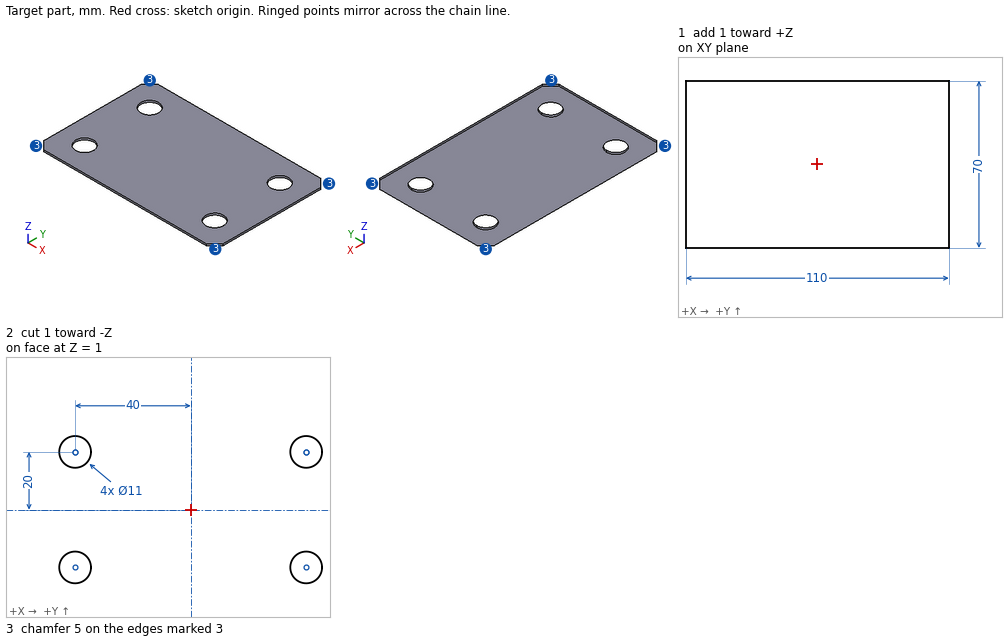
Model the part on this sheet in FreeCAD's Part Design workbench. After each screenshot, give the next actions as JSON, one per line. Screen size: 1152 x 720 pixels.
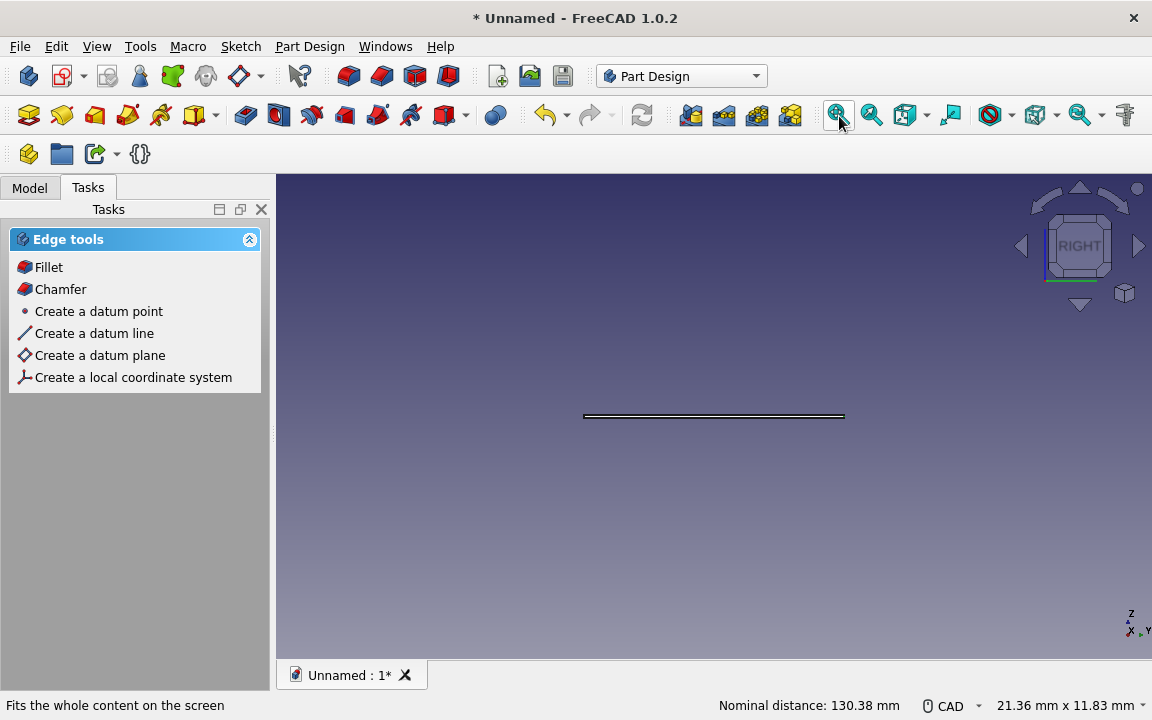
{"action": "key", "text": "5"}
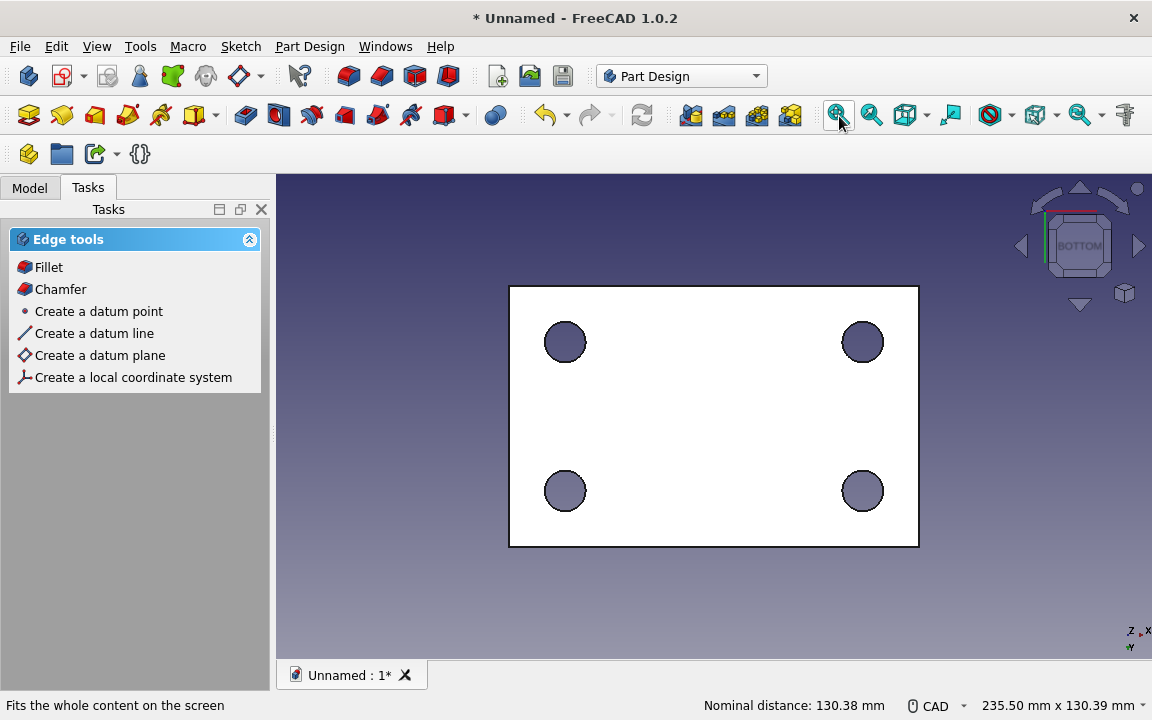
{"action": "scroll", "coordinate": [509, 546], "scroll_direction": "up", "scroll_amount": 12}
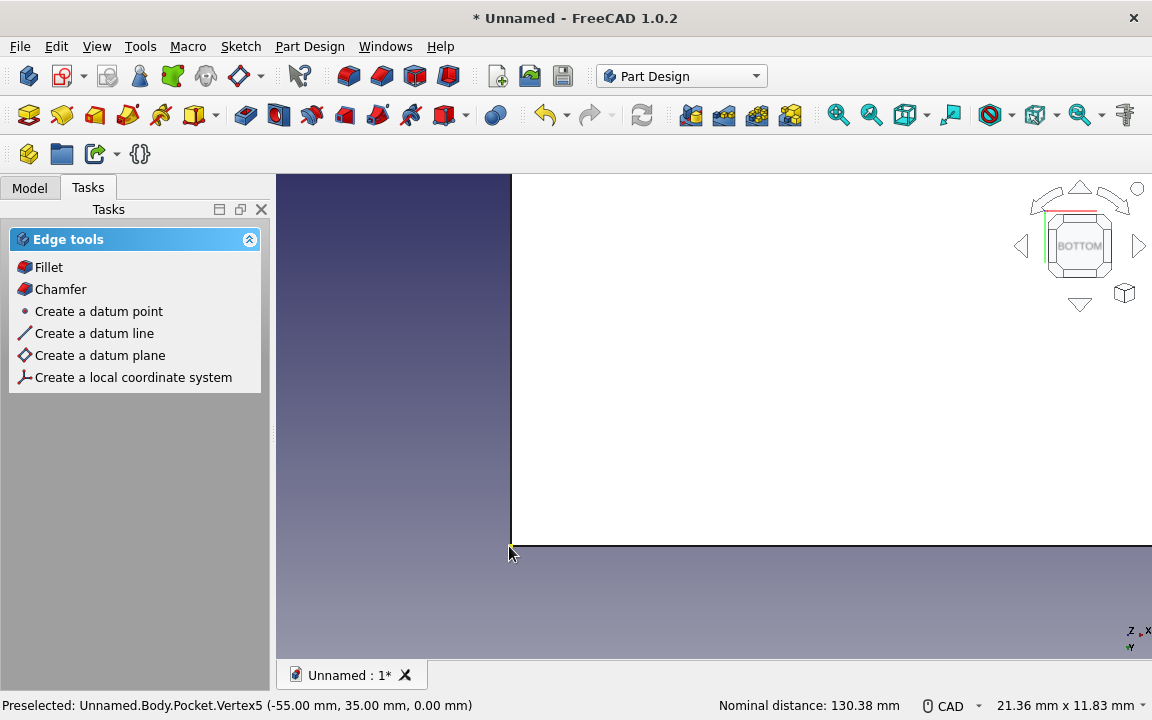
{"action": "left_click", "coordinate": [839, 116]}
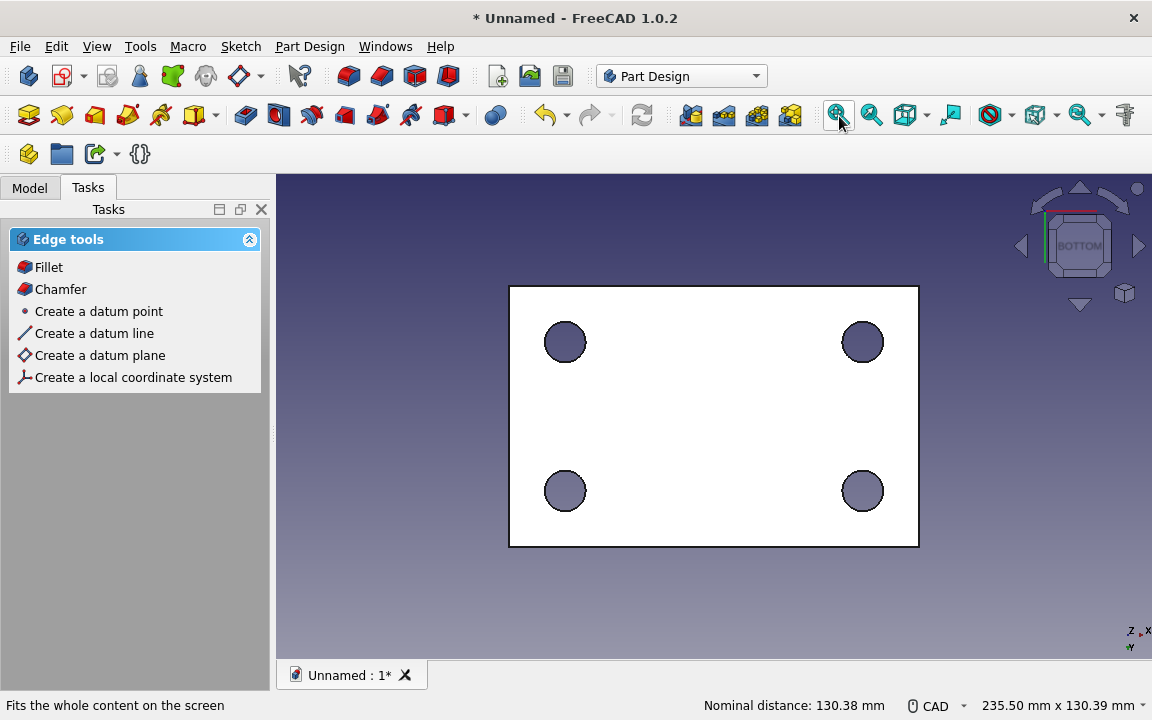
{"action": "key", "text": "4"}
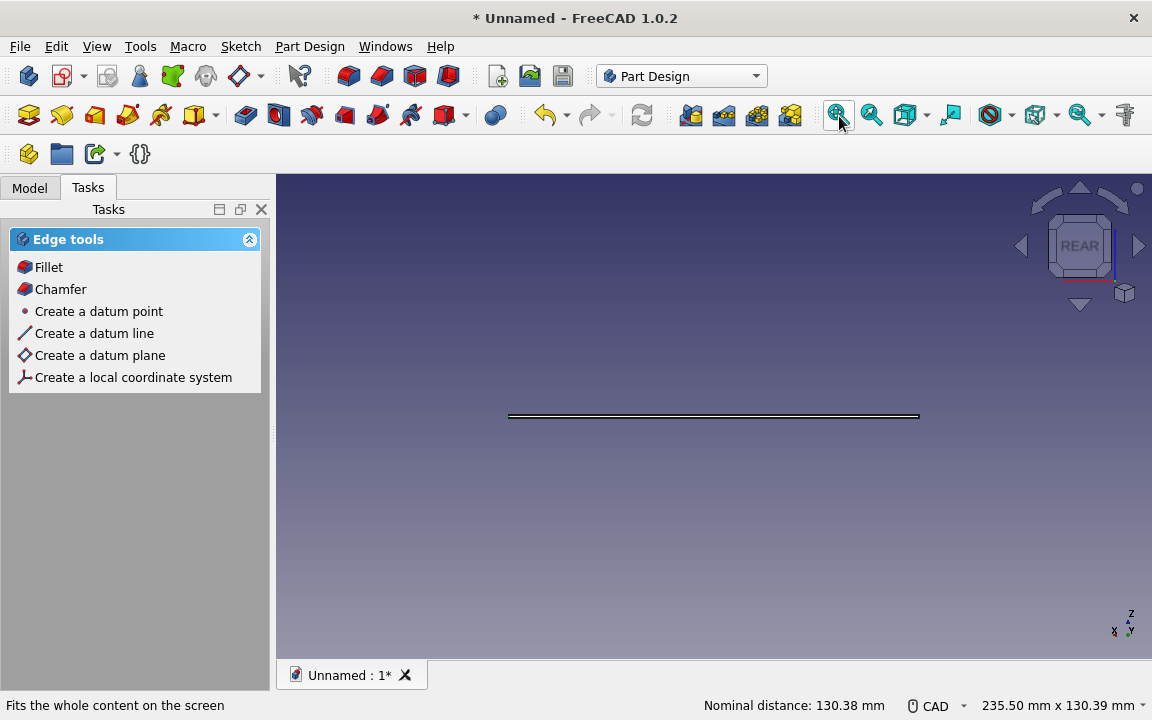
{"action": "scroll", "coordinate": [919, 415], "scroll_direction": "up", "scroll_amount": 12}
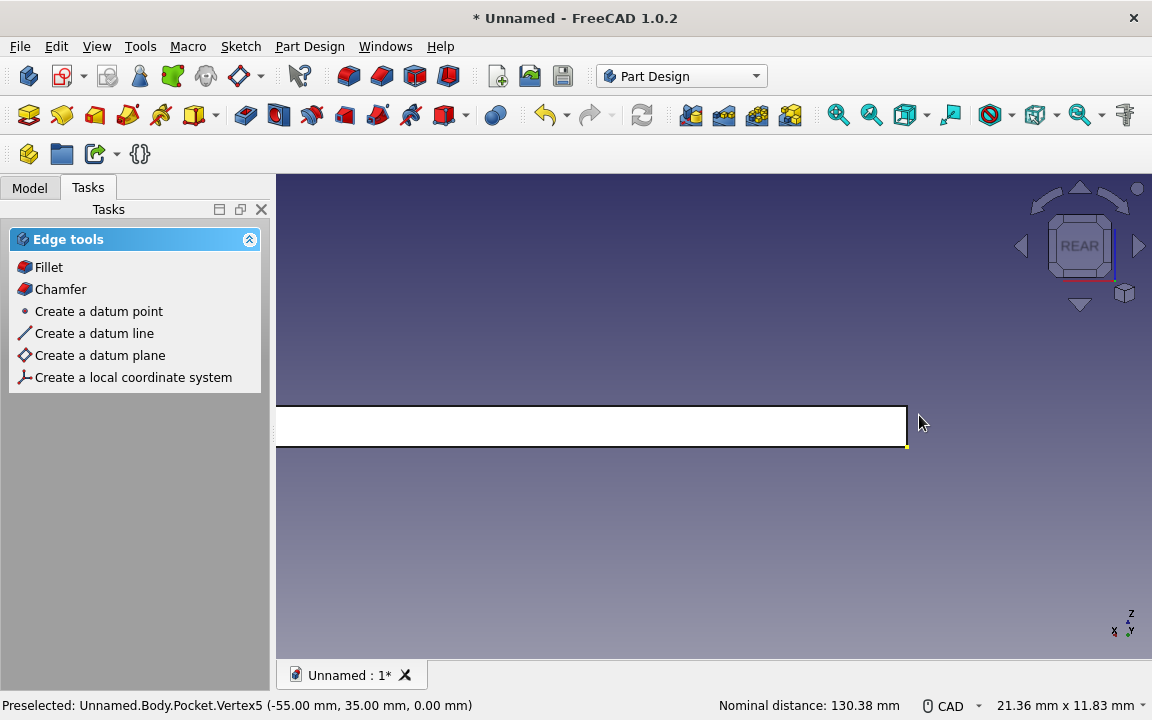
{"action": "left_click", "coordinate": [907, 426], "text": "ctrl"}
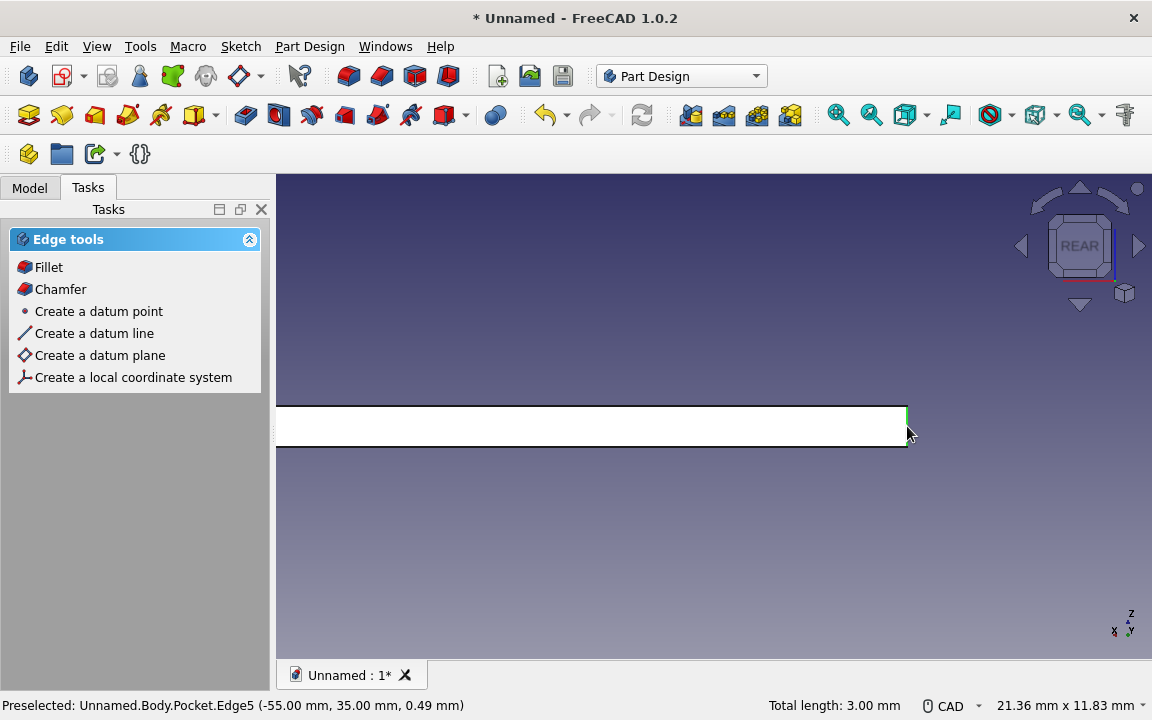
{"action": "left_click", "coordinate": [839, 116]}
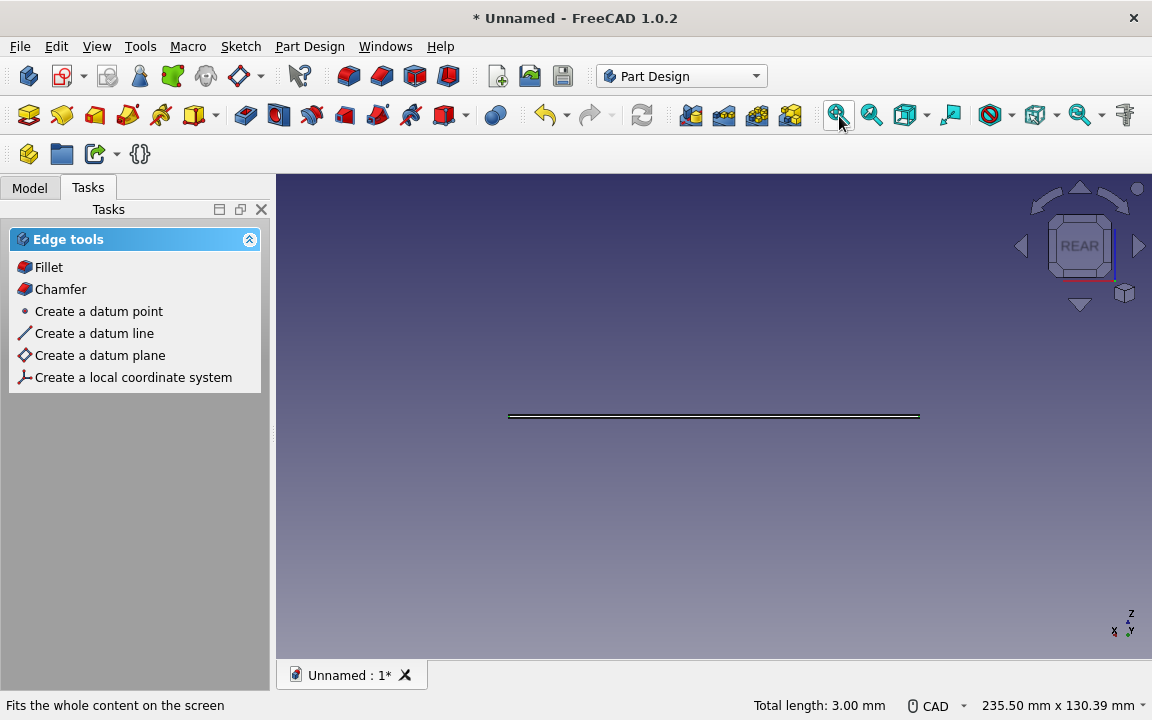
{"action": "key", "text": "6"}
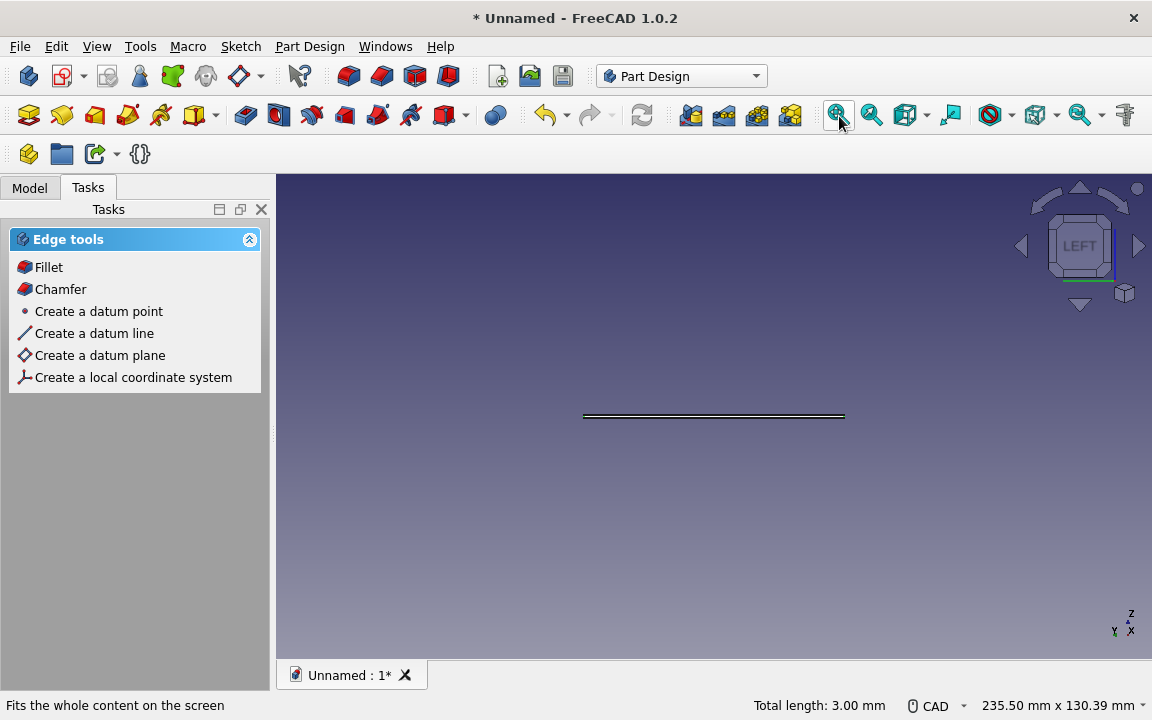
{"action": "left_click", "coordinate": [839, 116]}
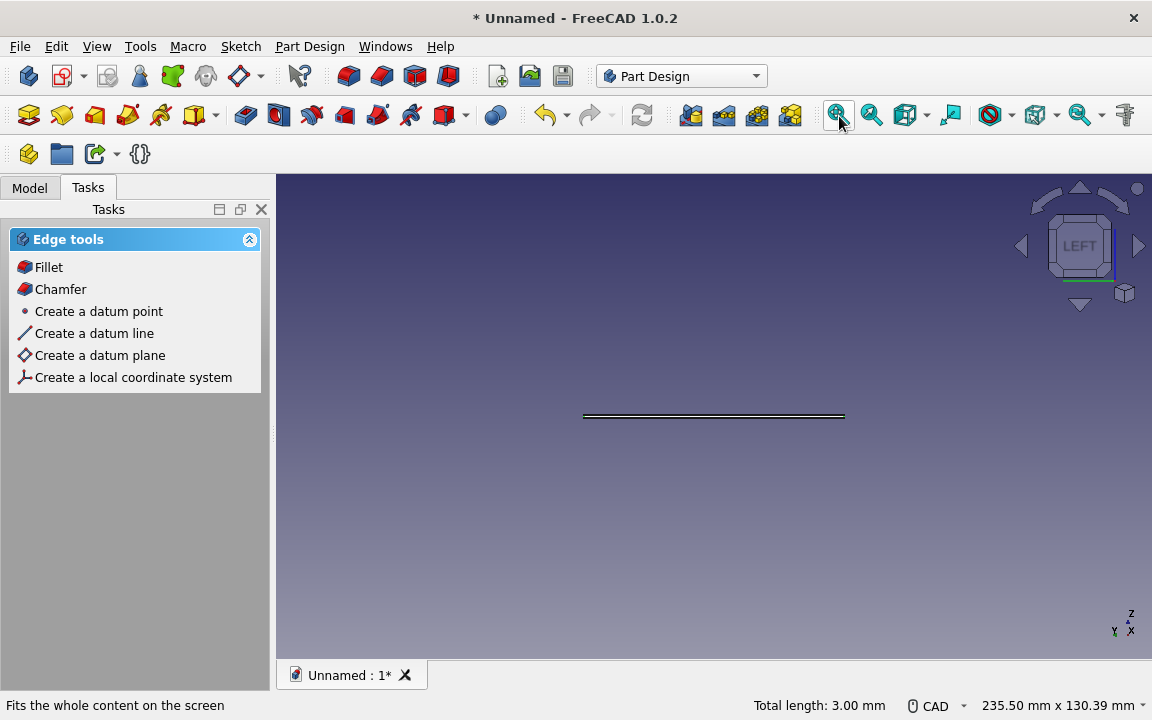
{"action": "scroll", "coordinate": [844, 415], "scroll_direction": "up", "scroll_amount": 12}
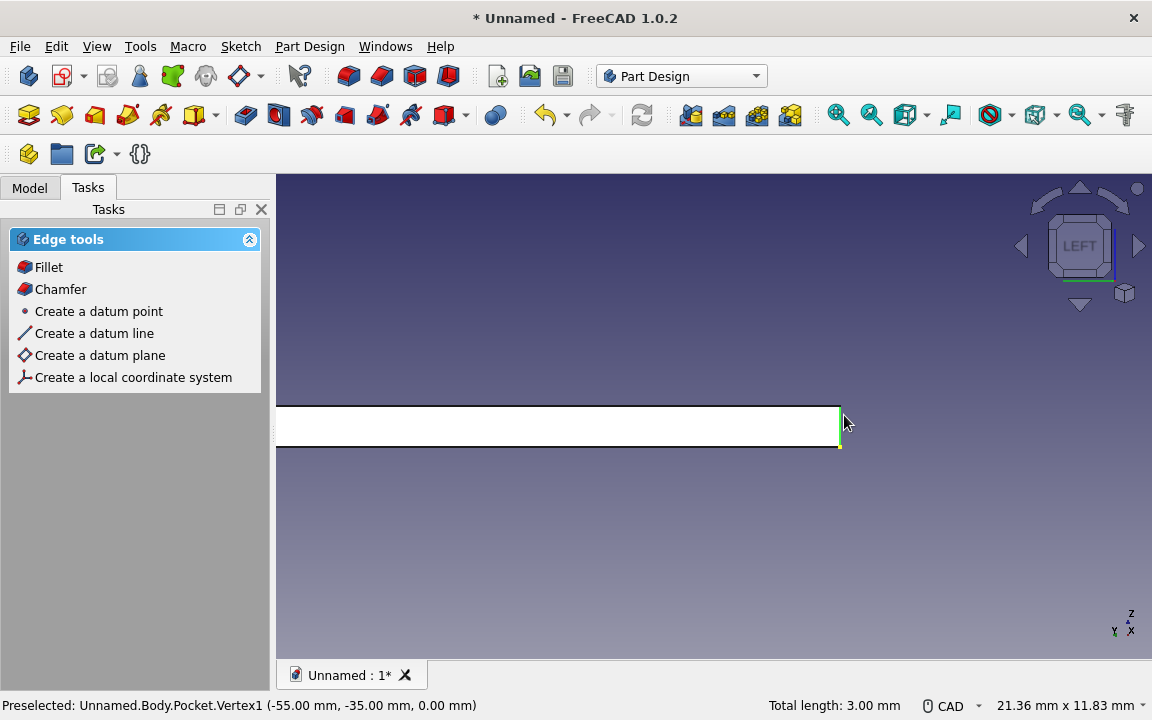
{"action": "left_click", "coordinate": [839, 116]}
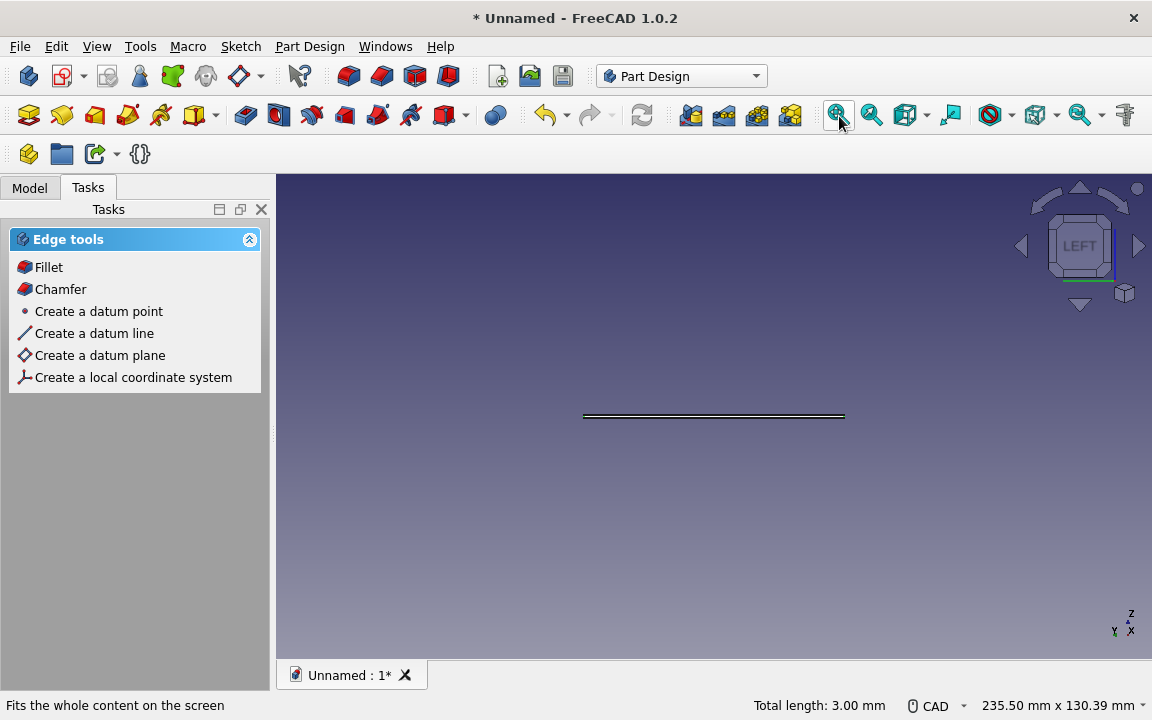
{"action": "key", "text": "v 3"}